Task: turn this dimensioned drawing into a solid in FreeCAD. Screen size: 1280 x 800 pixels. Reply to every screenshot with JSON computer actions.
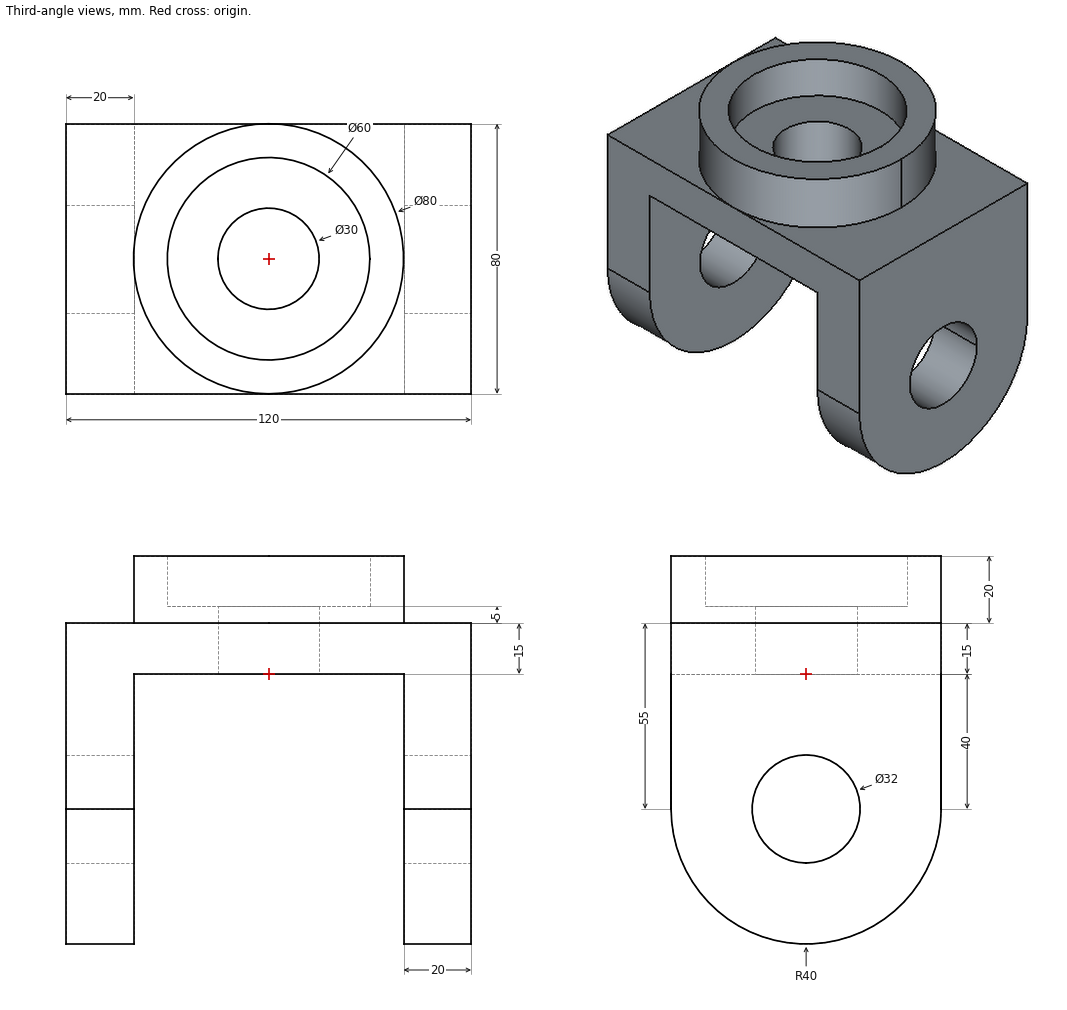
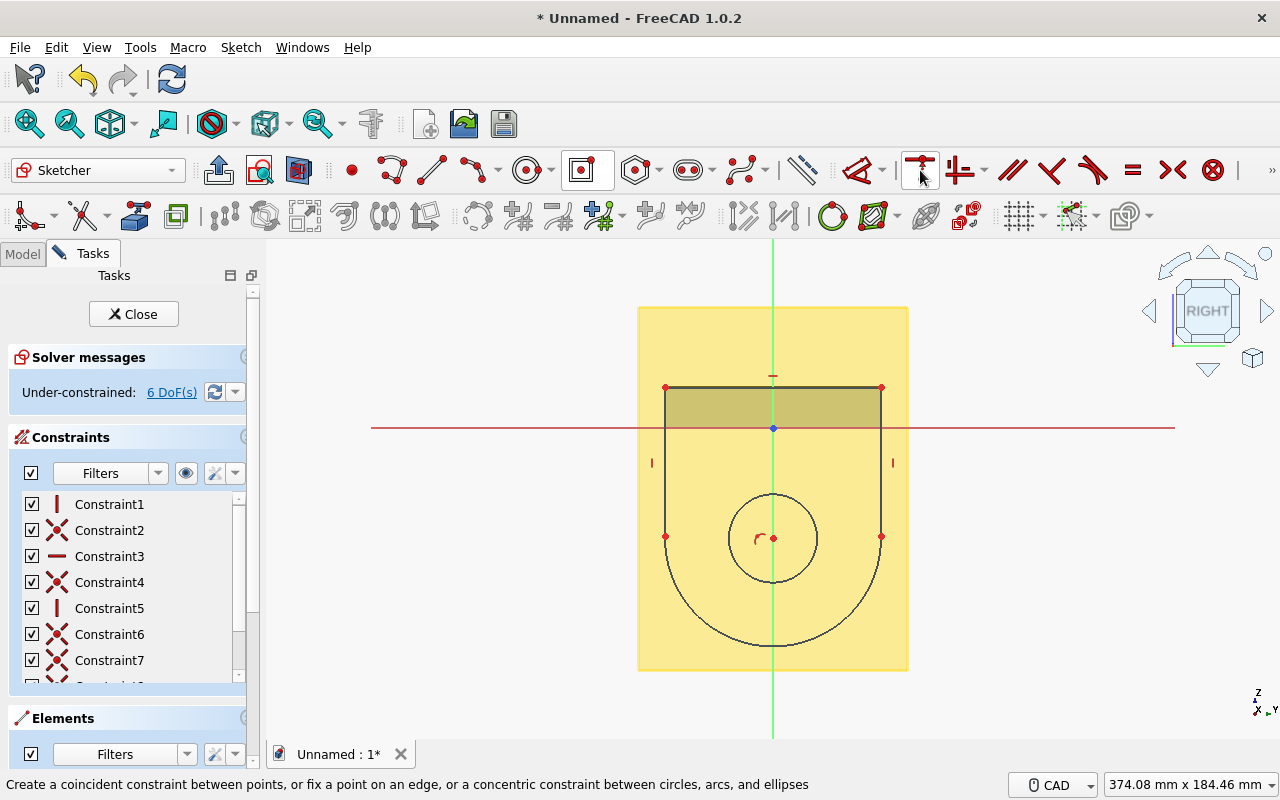
{"action": "left_click", "coordinate": [858, 170]}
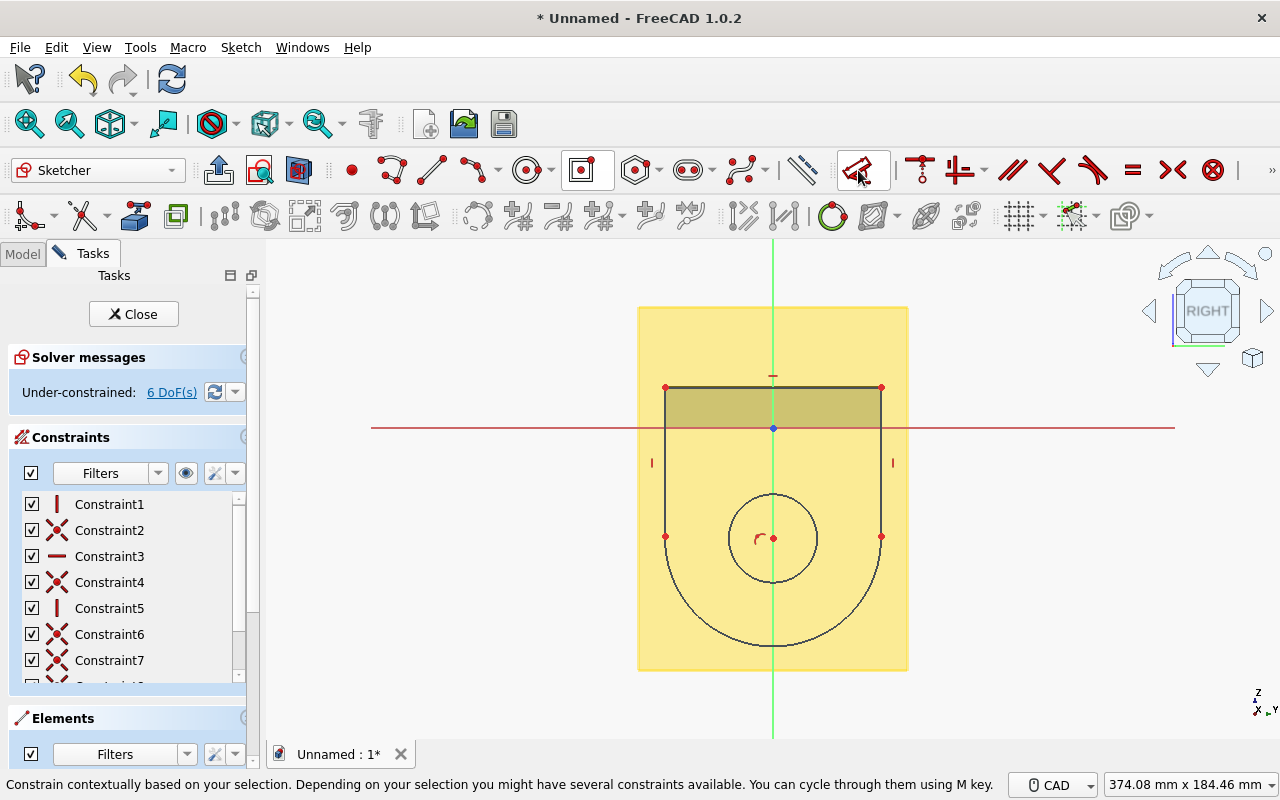
{"action": "left_click", "coordinate": [709, 626]}
{"action": "left_click", "coordinate": [690, 652]}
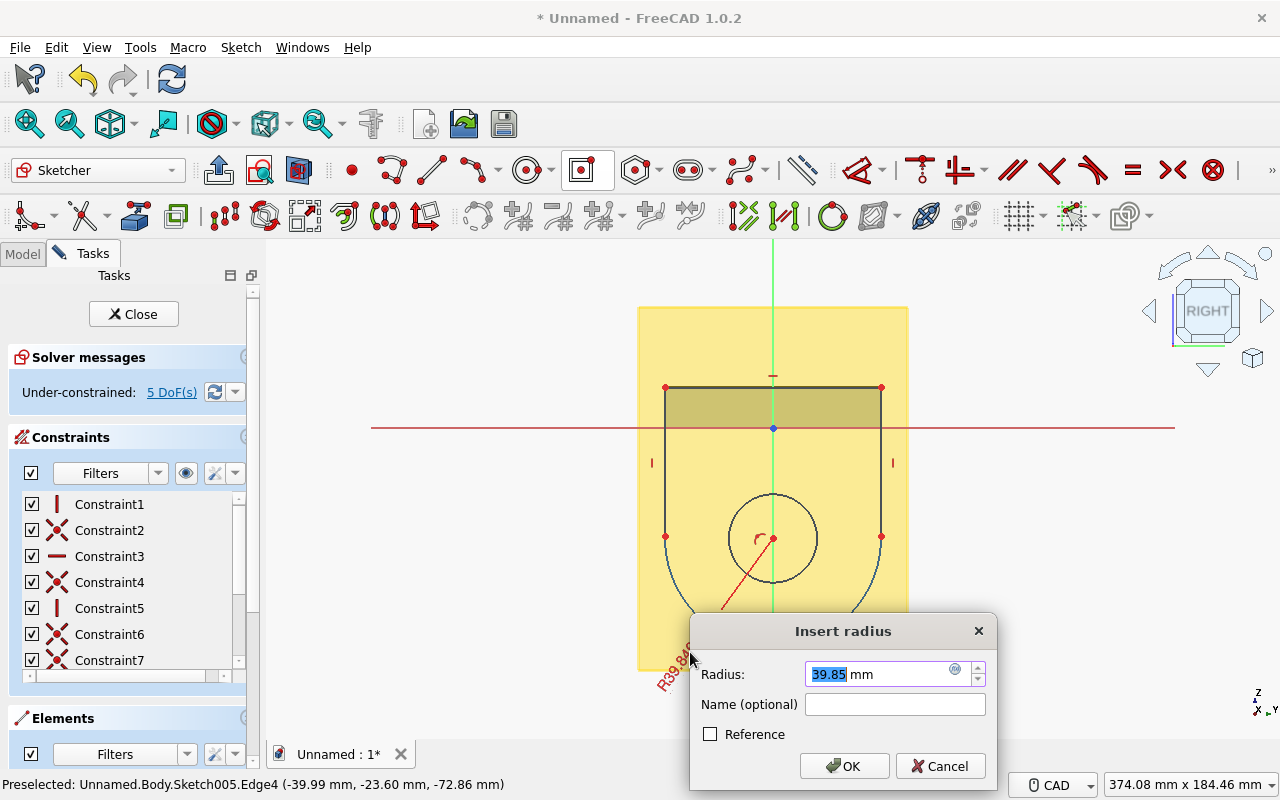
{"action": "type", "text": "40"}
{"action": "key", "text": "Return"}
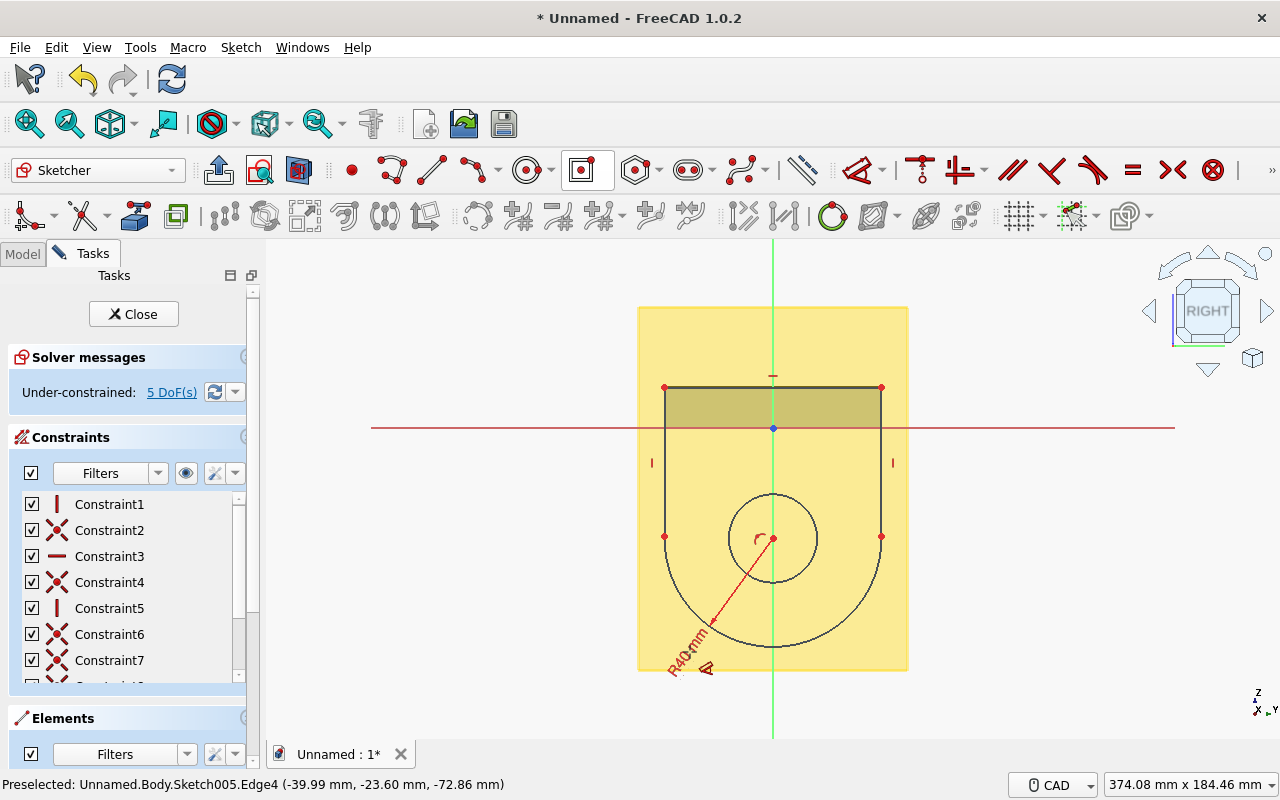
{"action": "left_click", "coordinate": [804, 507]}
{"action": "left_click", "coordinate": [826, 484]}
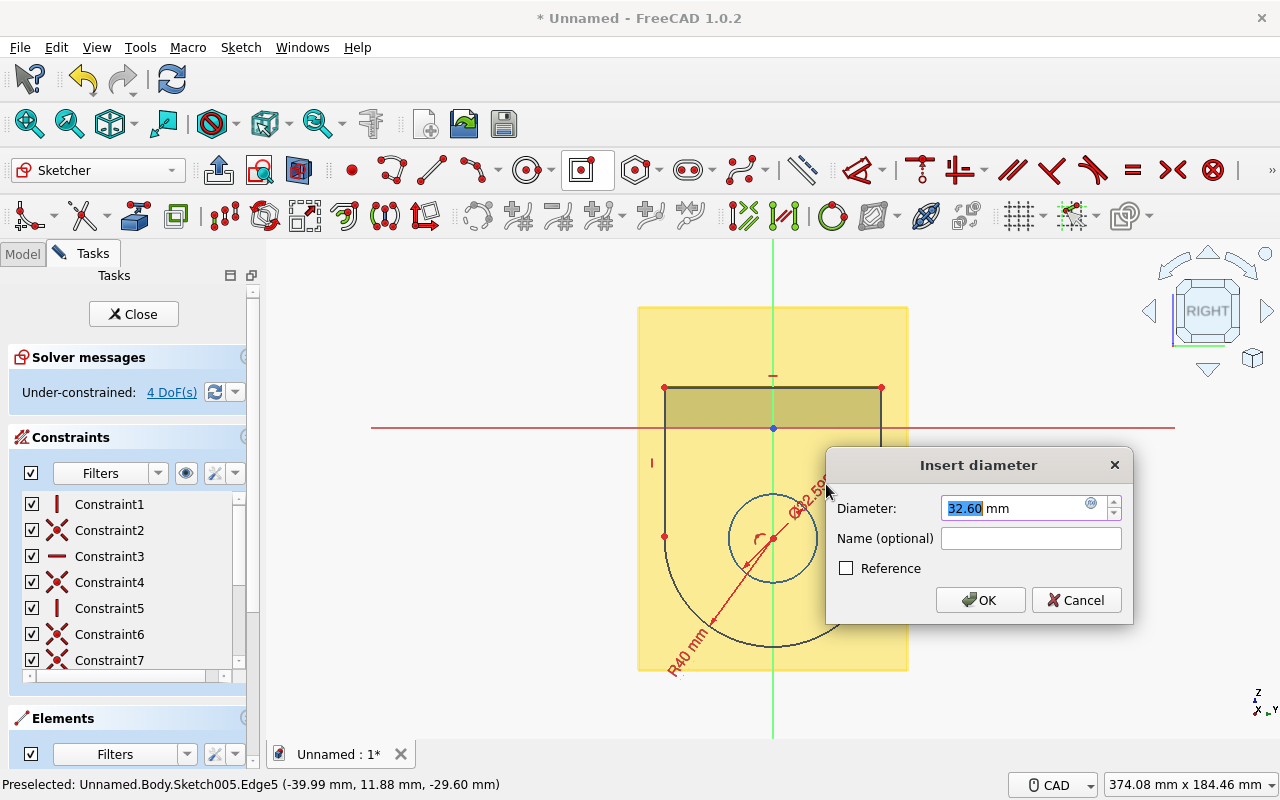
{"action": "type", "text": "32"}
{"action": "key", "text": "Return"}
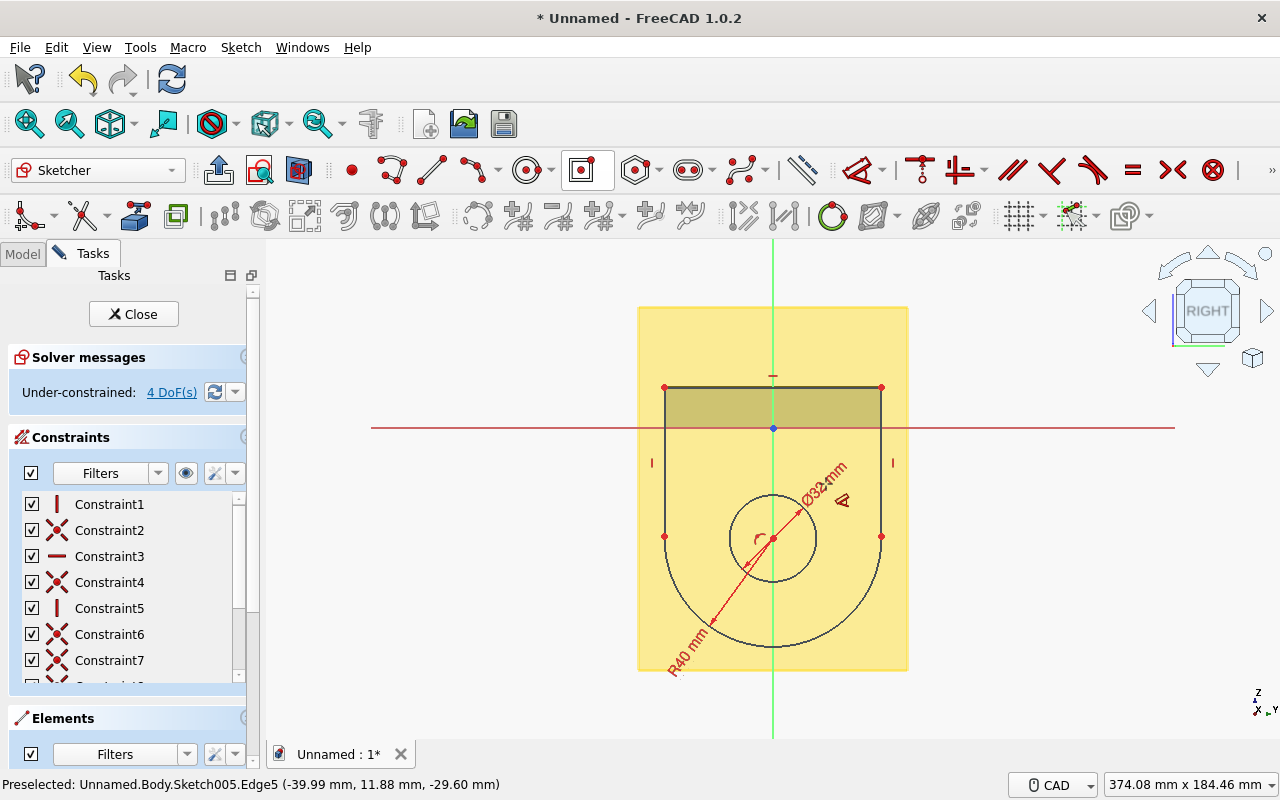
{"action": "left_click", "coordinate": [665, 492]}
{"action": "left_click", "coordinate": [631, 463]}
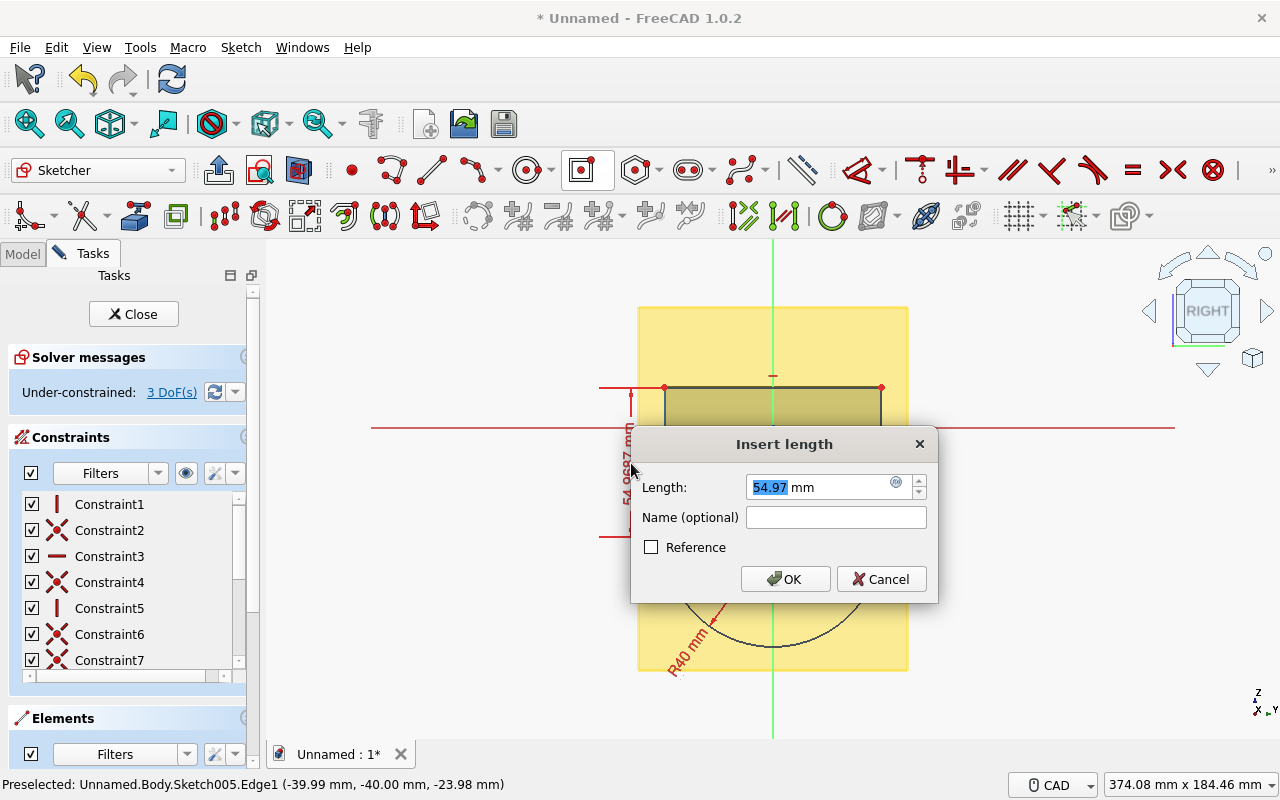
{"action": "type", "text": "55"}
{"action": "key", "text": "Return"}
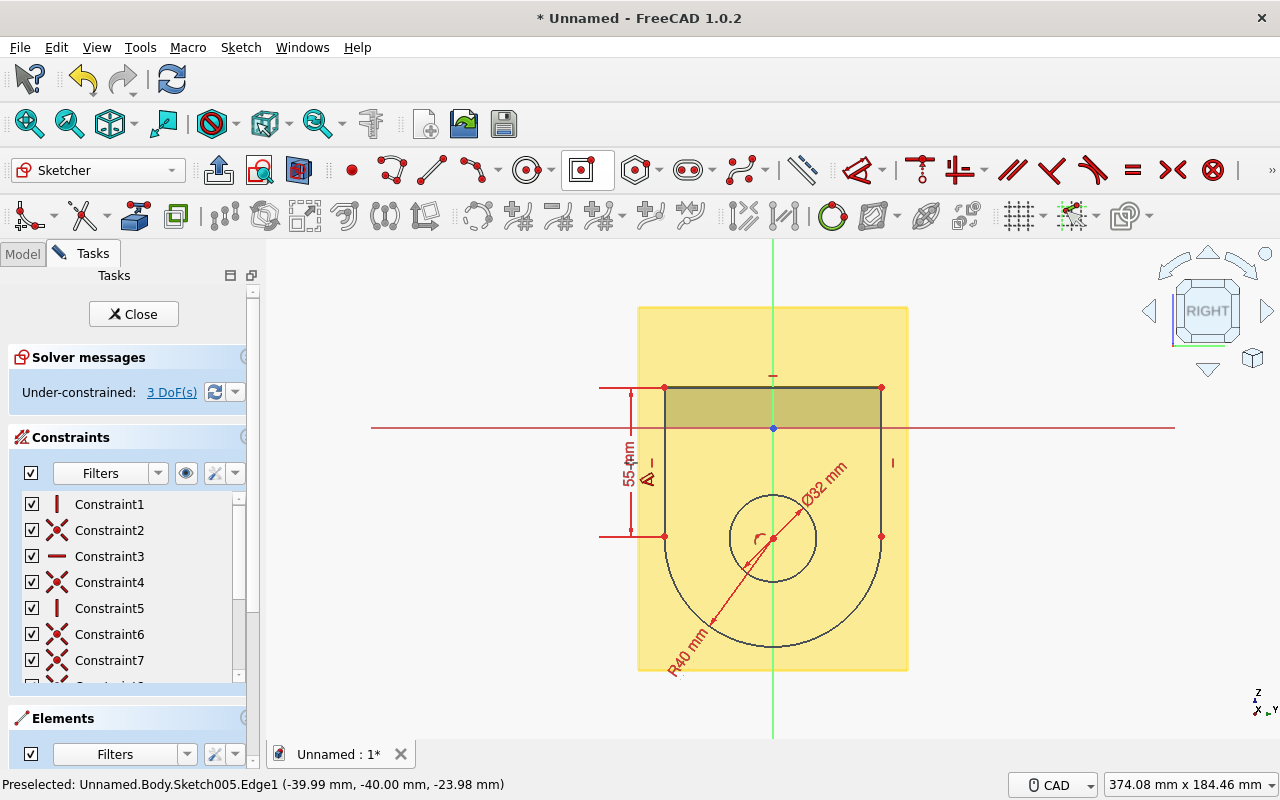
{"action": "left_click", "coordinate": [881, 492]}
{"action": "left_click", "coordinate": [915, 462]}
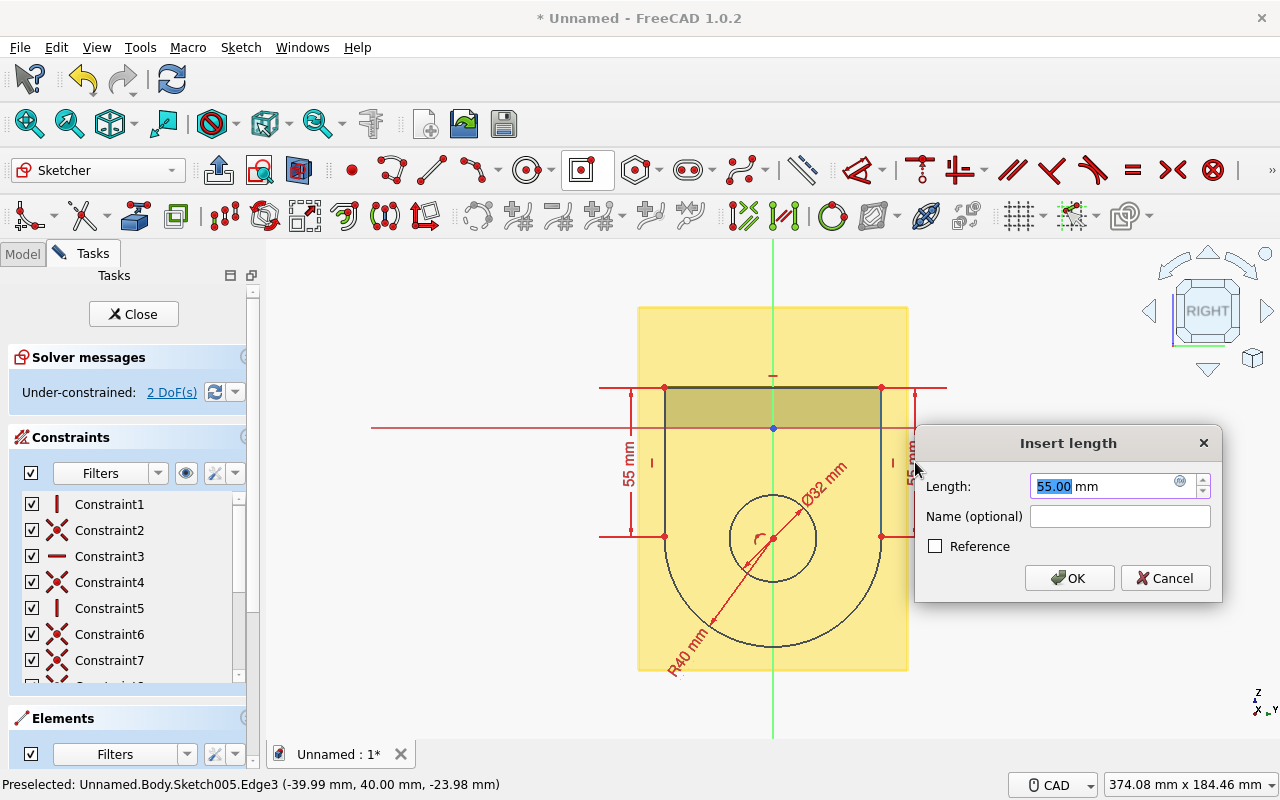
{"action": "type", "text": "55"}
{"action": "key", "text": "Return"}